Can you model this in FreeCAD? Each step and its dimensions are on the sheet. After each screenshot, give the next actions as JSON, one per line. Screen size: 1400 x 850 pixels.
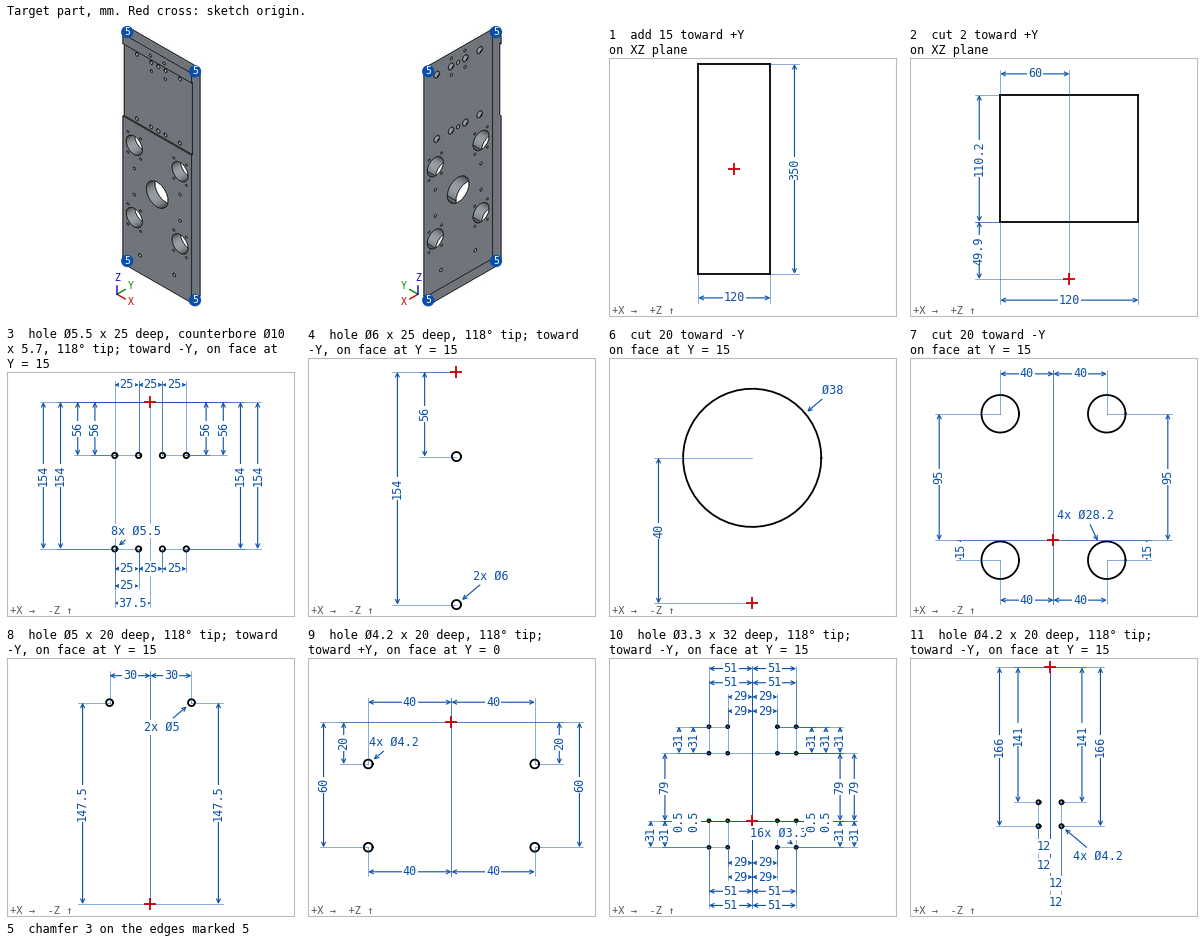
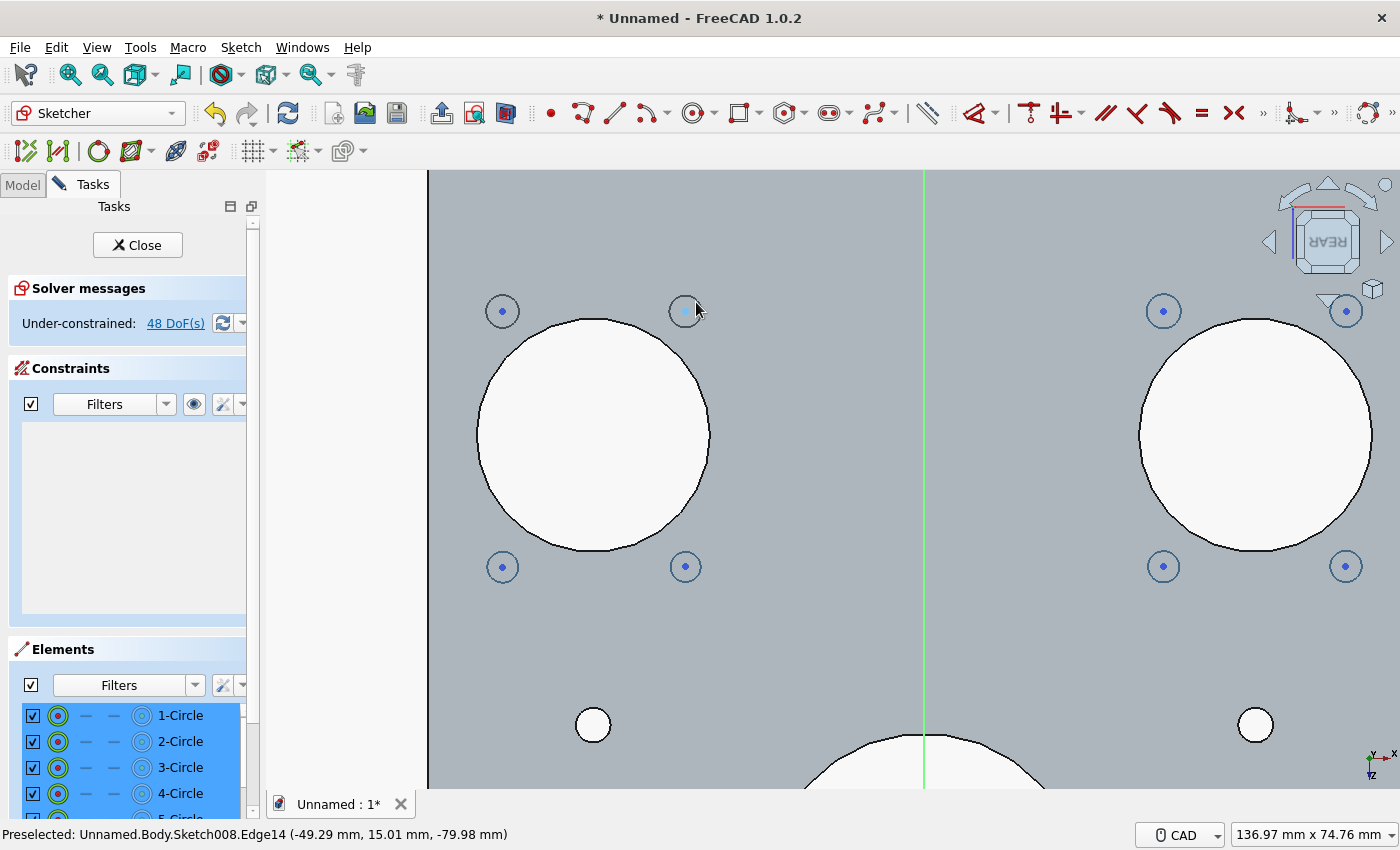
{"action": "left_click", "coordinate": [697, 300]}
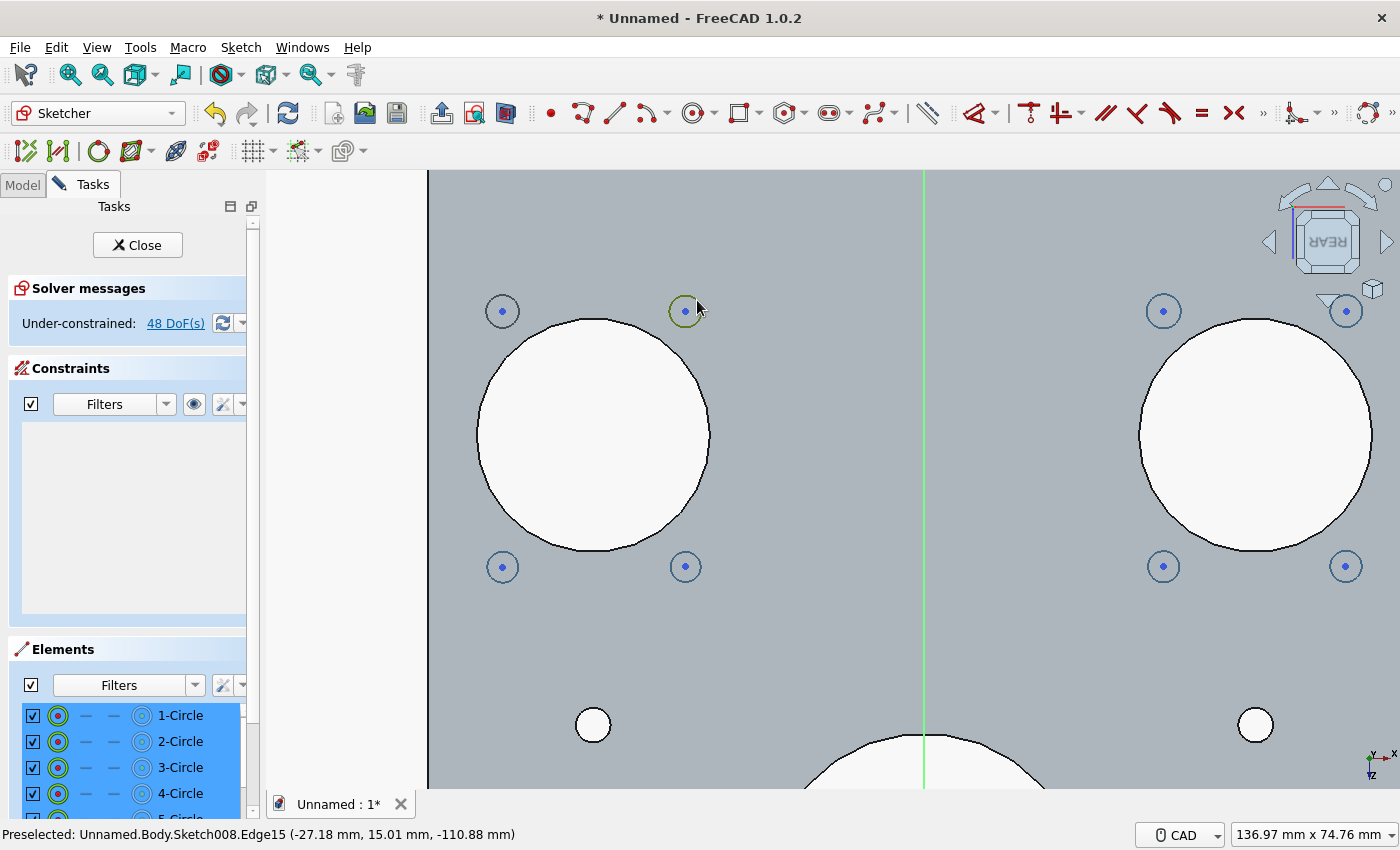
{"action": "left_click", "coordinate": [514, 300]}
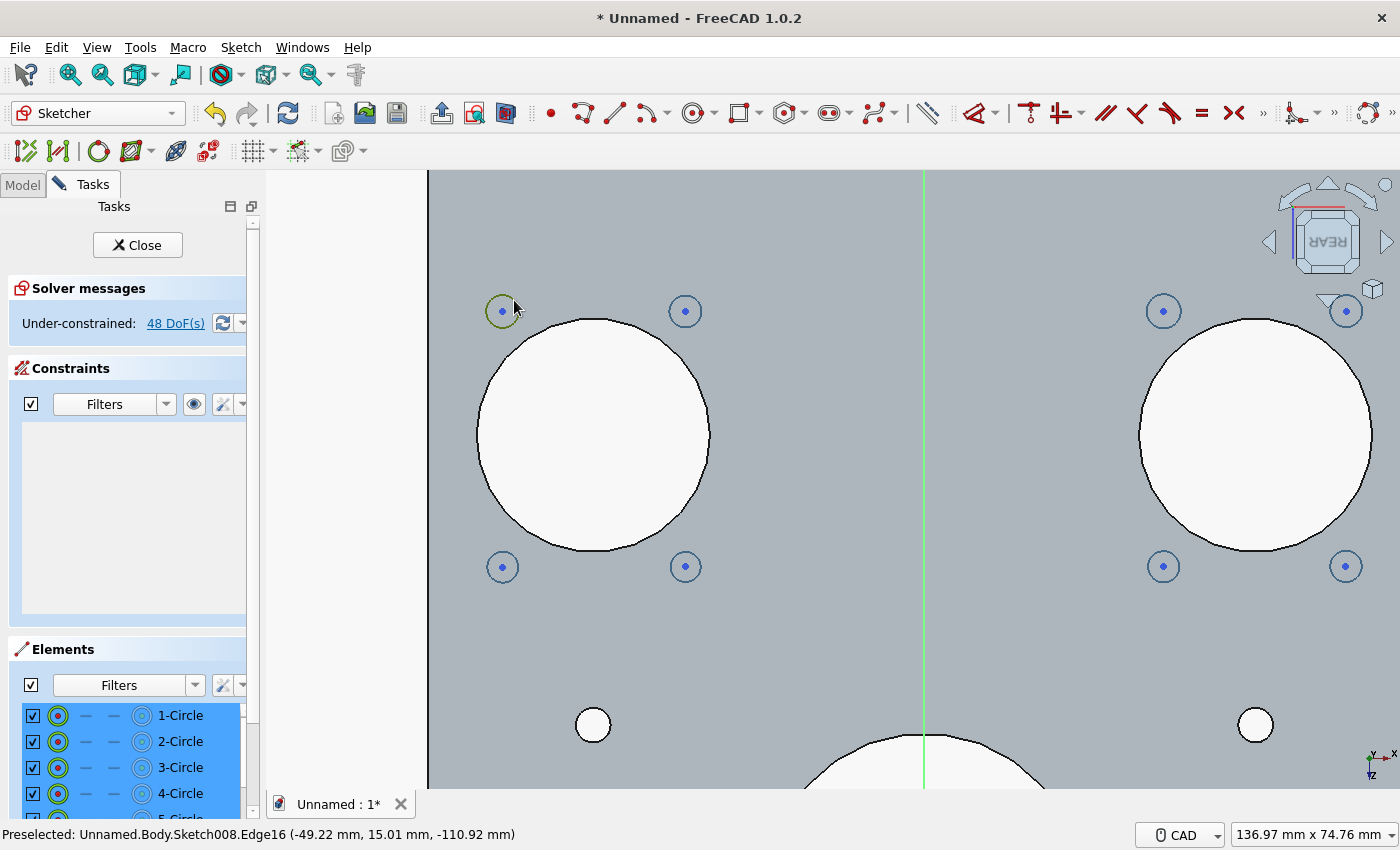
{"action": "left_click", "coordinate": [1202, 114]}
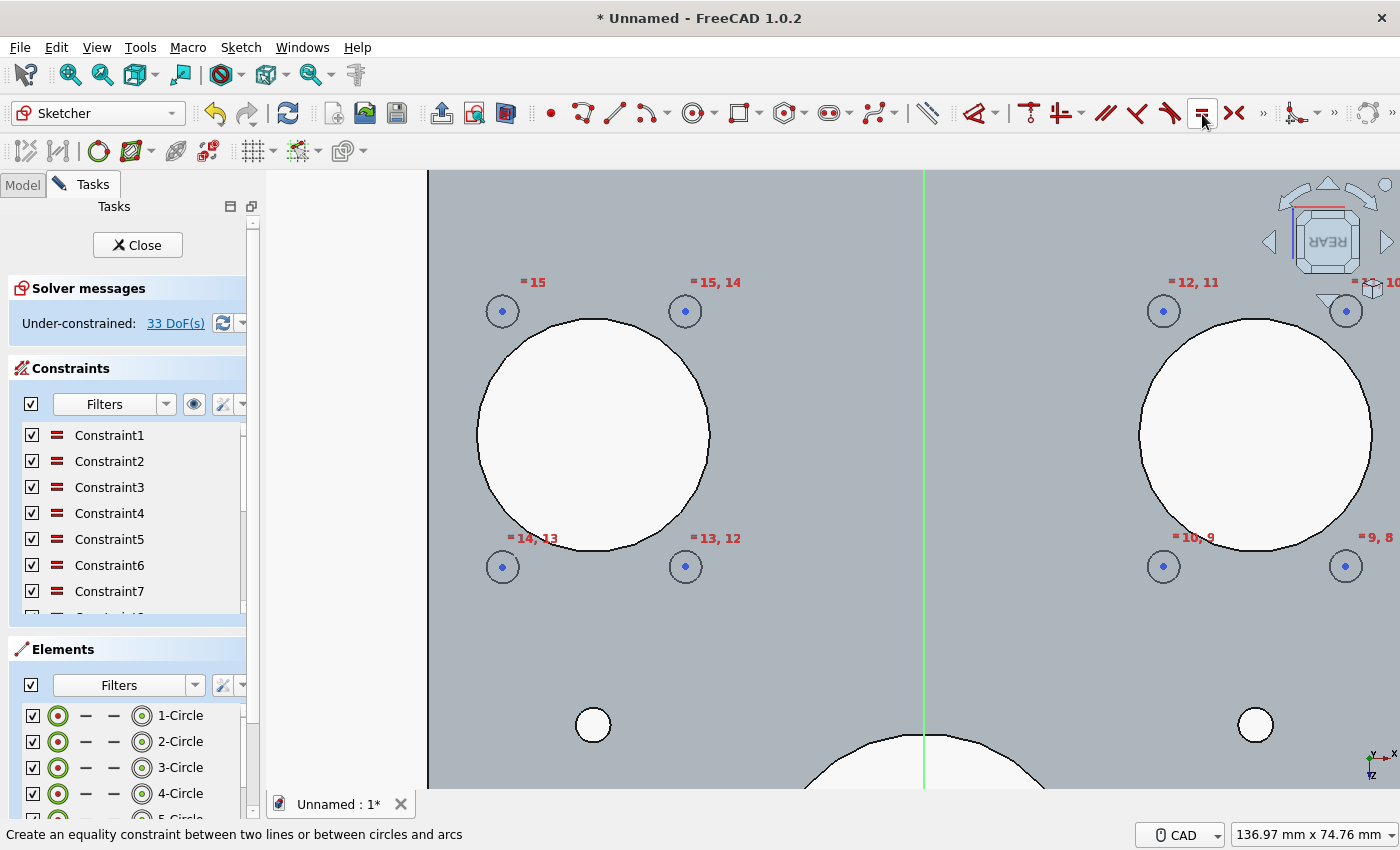
{"action": "left_click", "coordinate": [974, 114]}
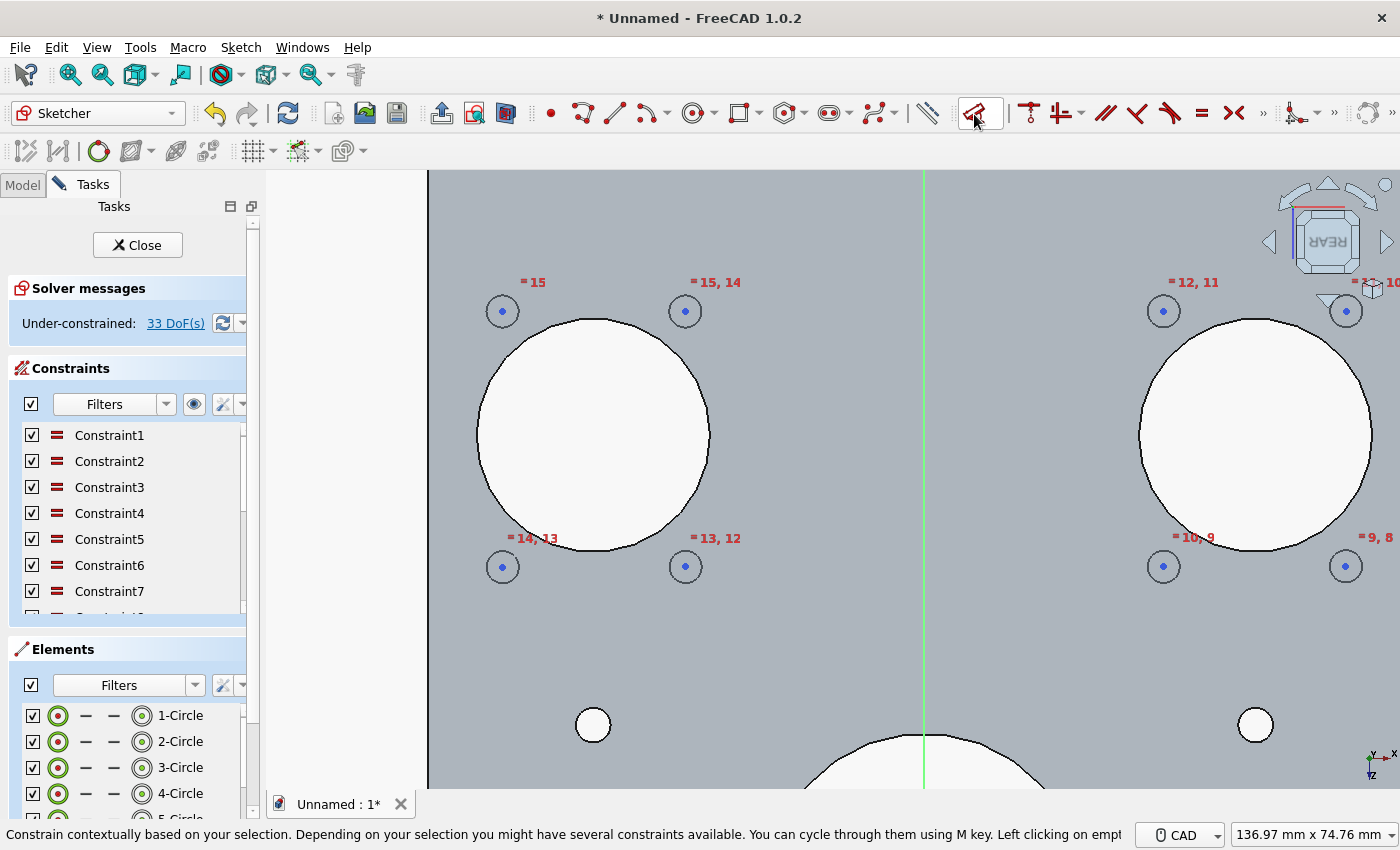
{"action": "scroll", "coordinate": [696, 302], "scroll_direction": "down", "scroll_amount": 6}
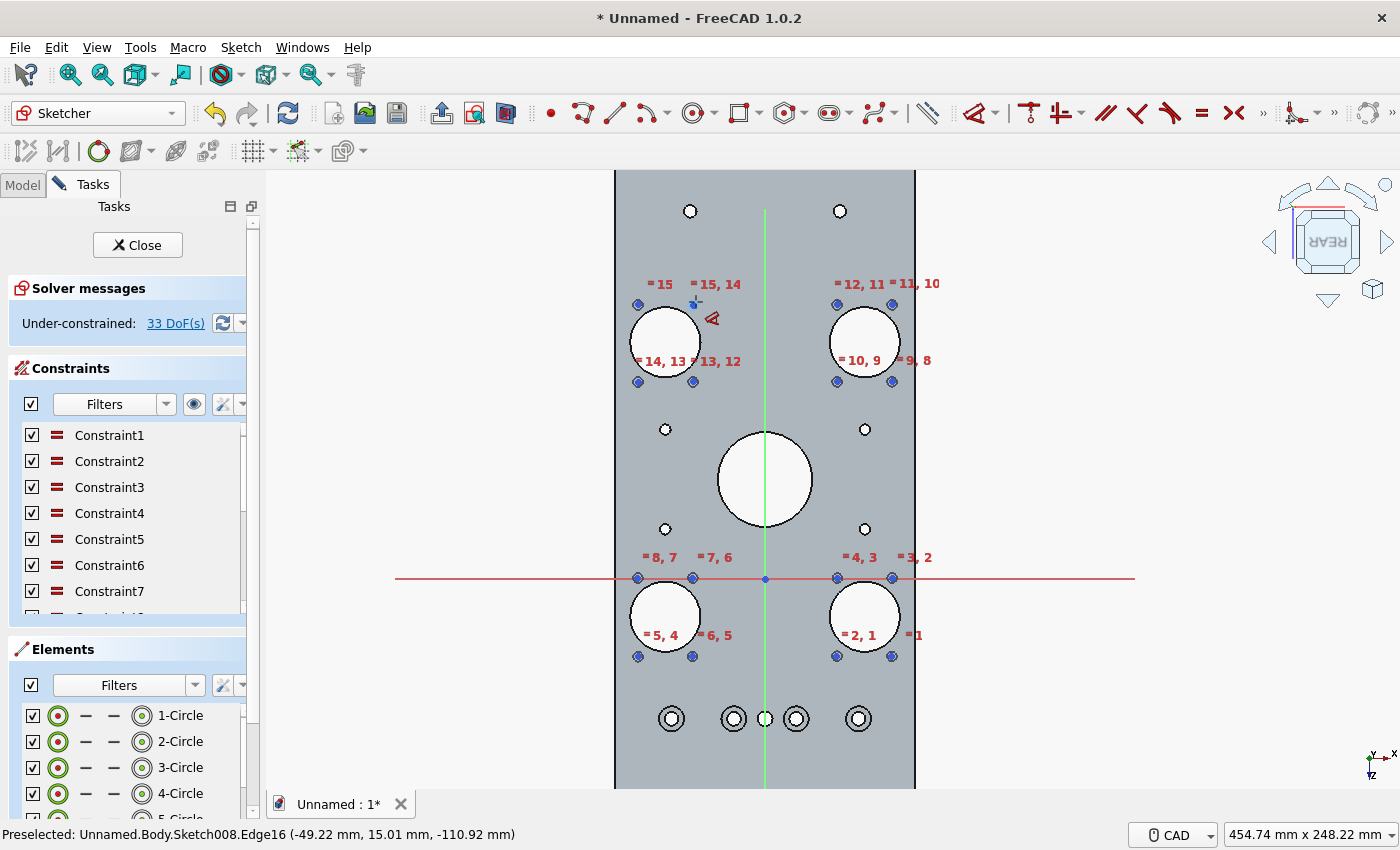
{"action": "scroll", "coordinate": [895, 653], "scroll_direction": "up", "scroll_amount": 8}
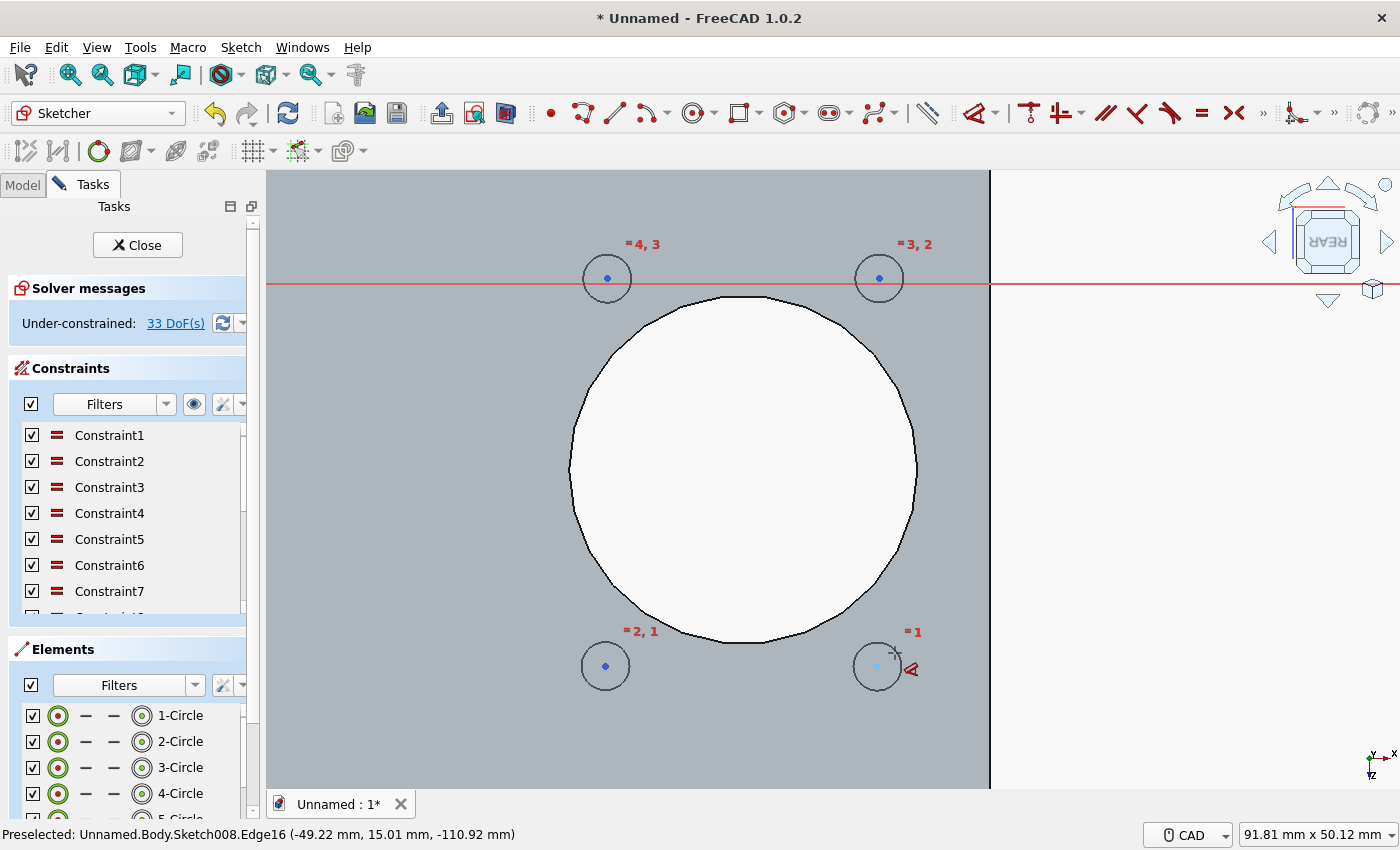
{"action": "left_click", "coordinate": [894, 650]}
{"action": "left_click", "coordinate": [917, 627]}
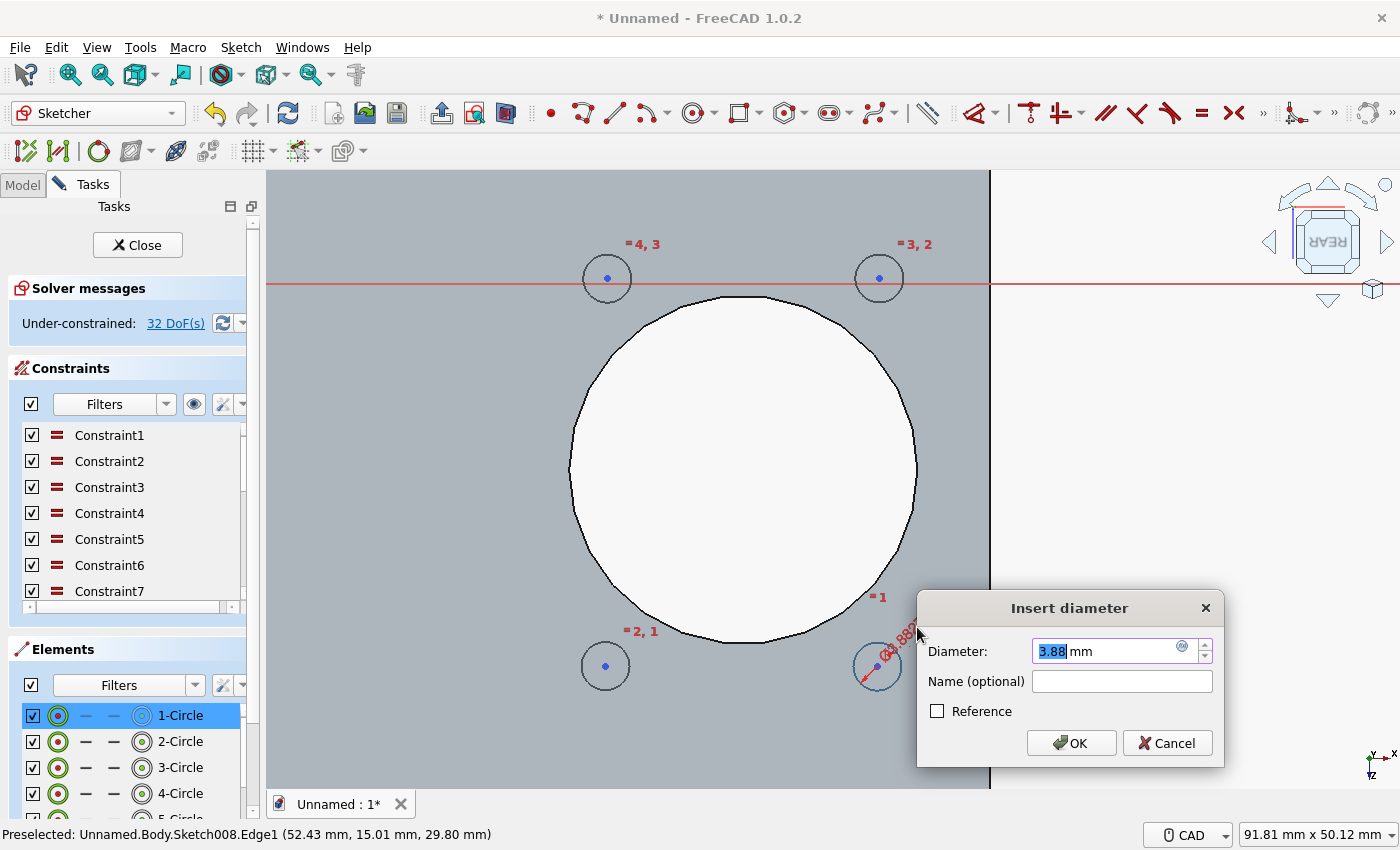
{"action": "type", "text": "3.3"}
{"action": "key", "text": "Return"}